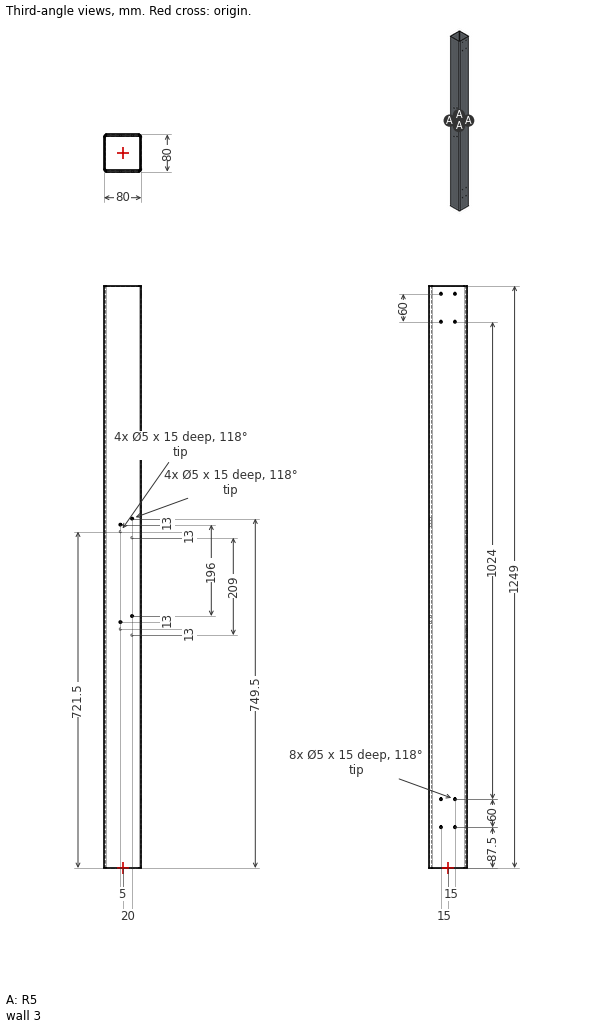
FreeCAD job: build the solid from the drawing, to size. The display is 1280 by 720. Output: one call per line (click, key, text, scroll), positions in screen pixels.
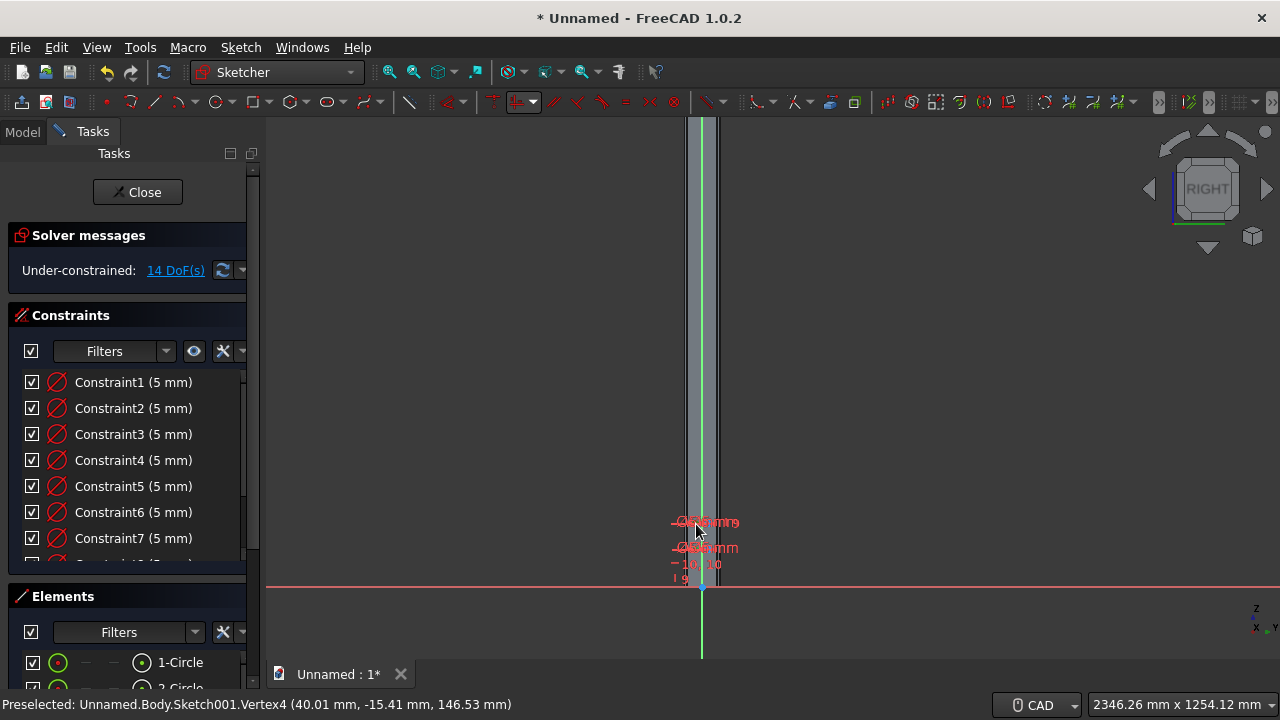
key(v)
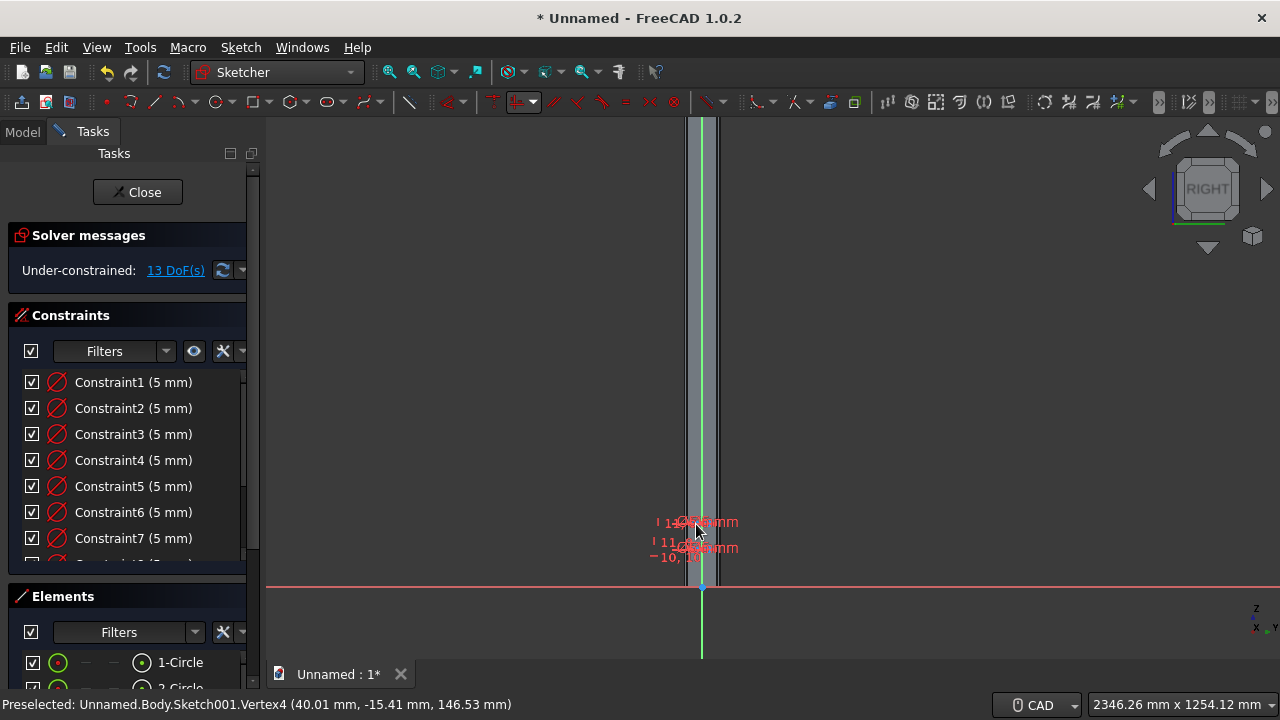
click(709, 524)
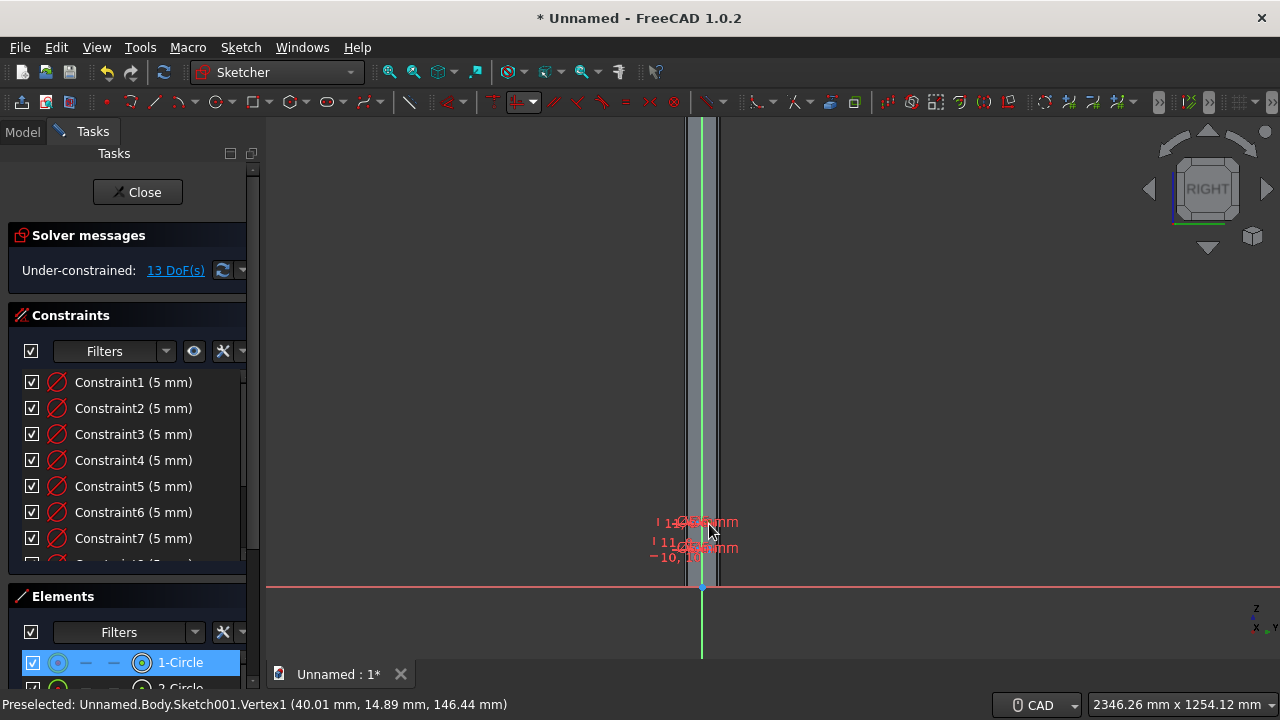
click(698, 526)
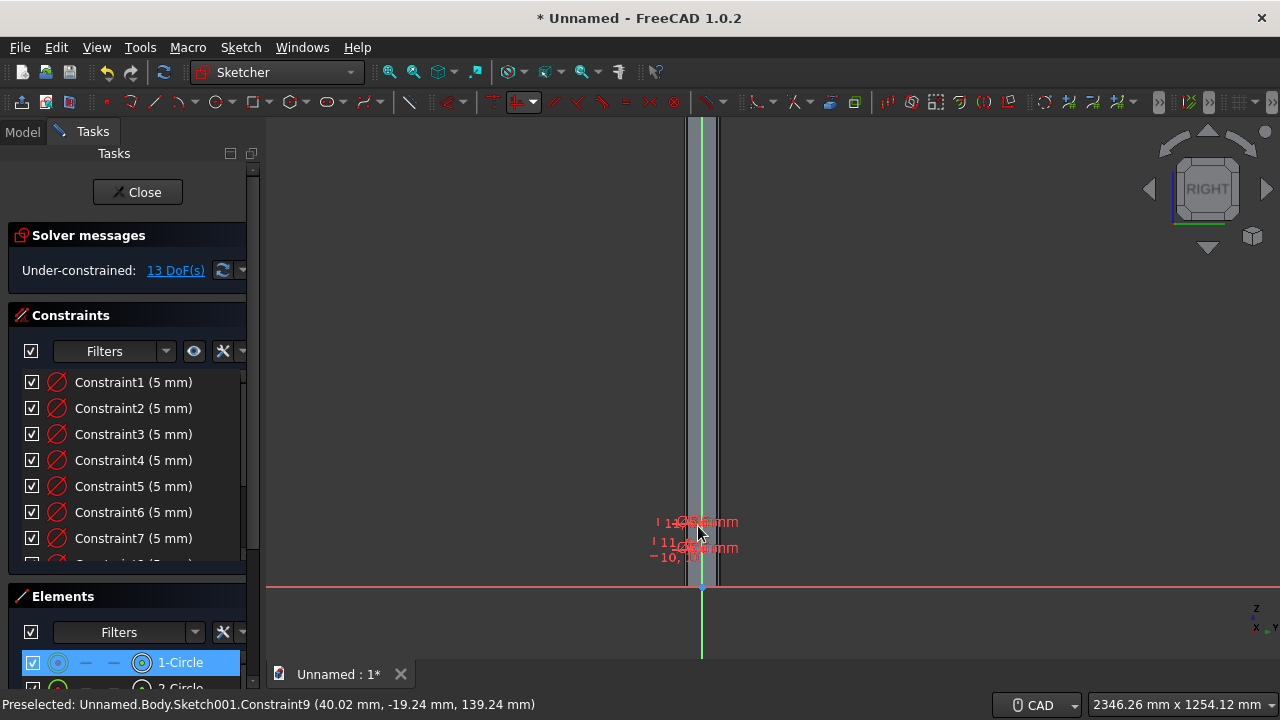
key(h)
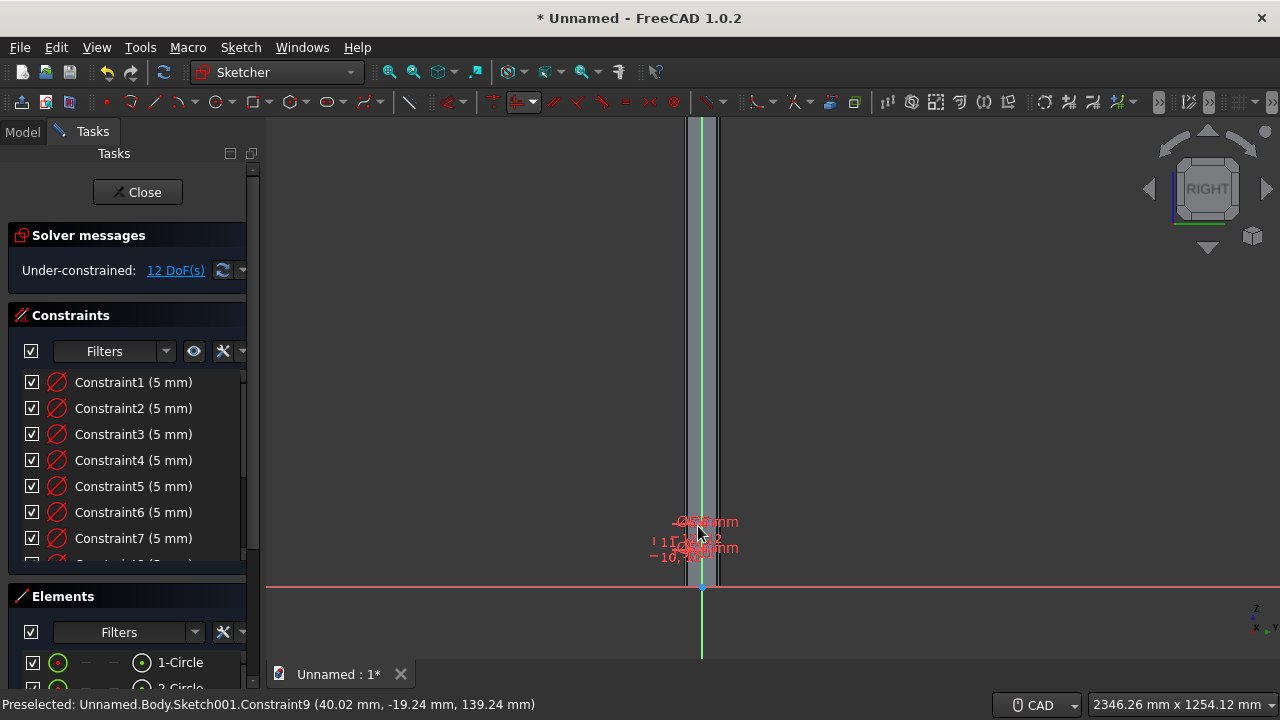
click(709, 524)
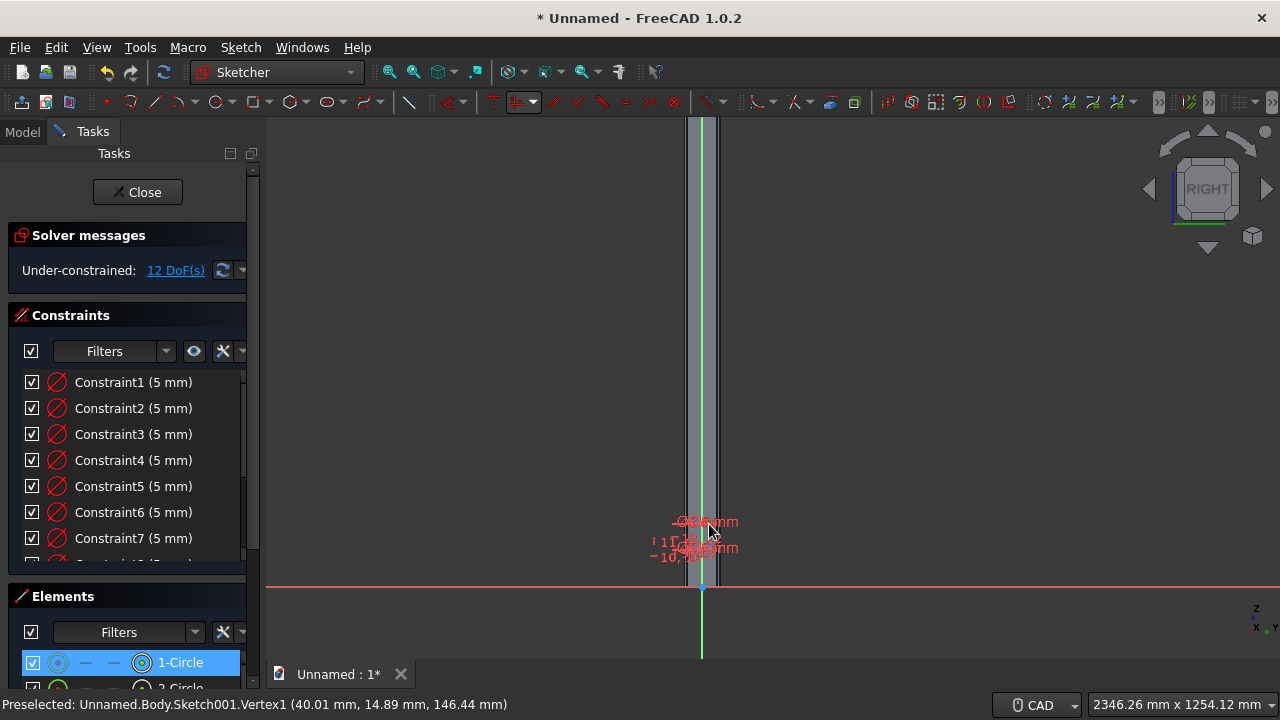
scroll(709, 525, down, 2)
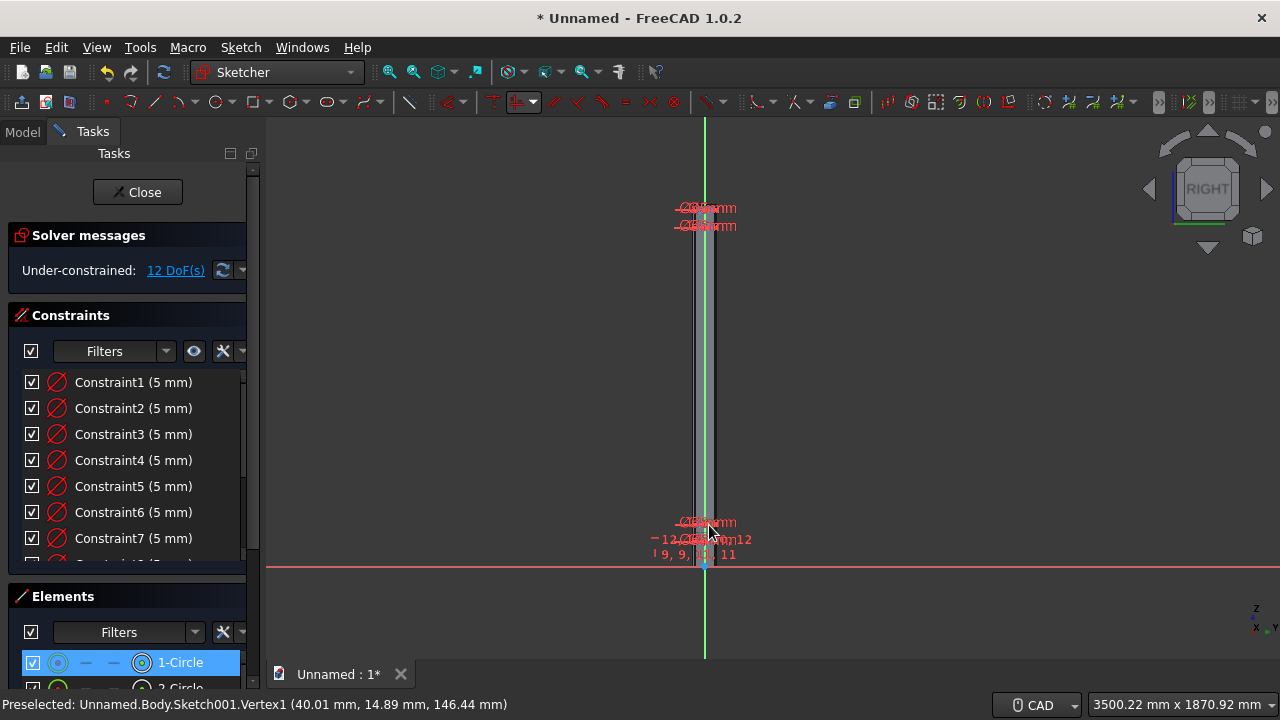
scroll(709, 228, up, 2)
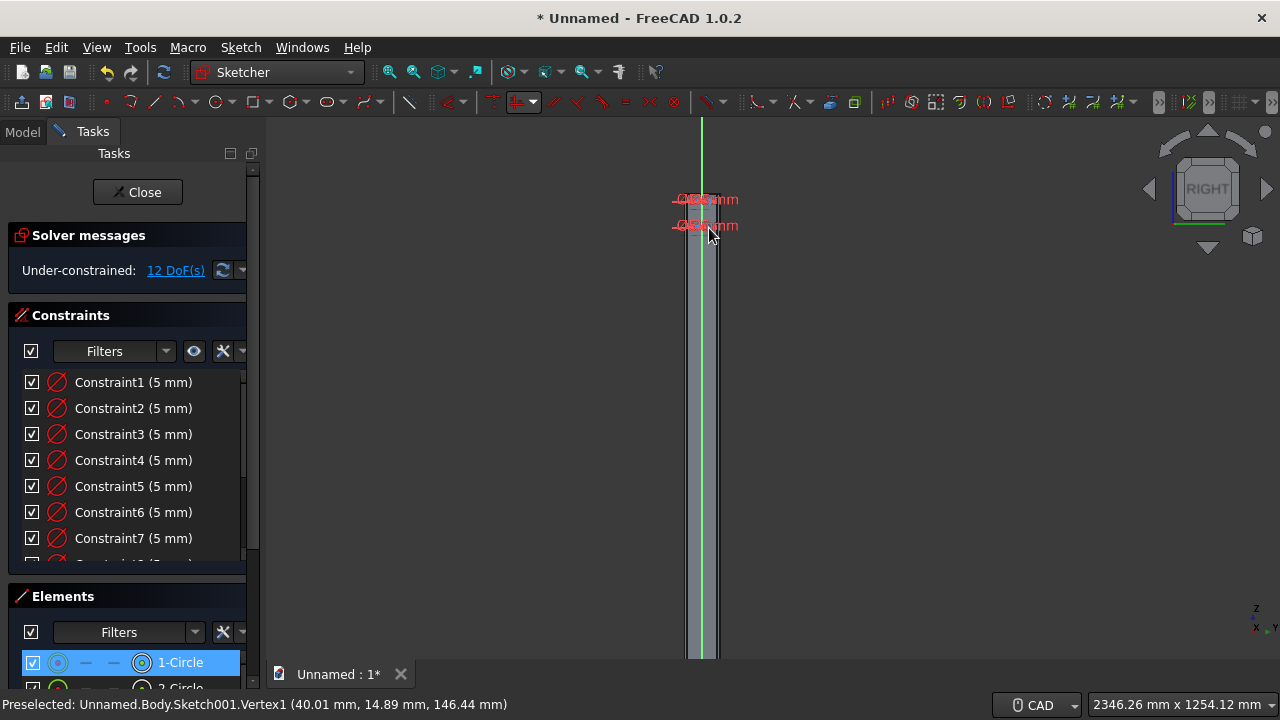
click(709, 228)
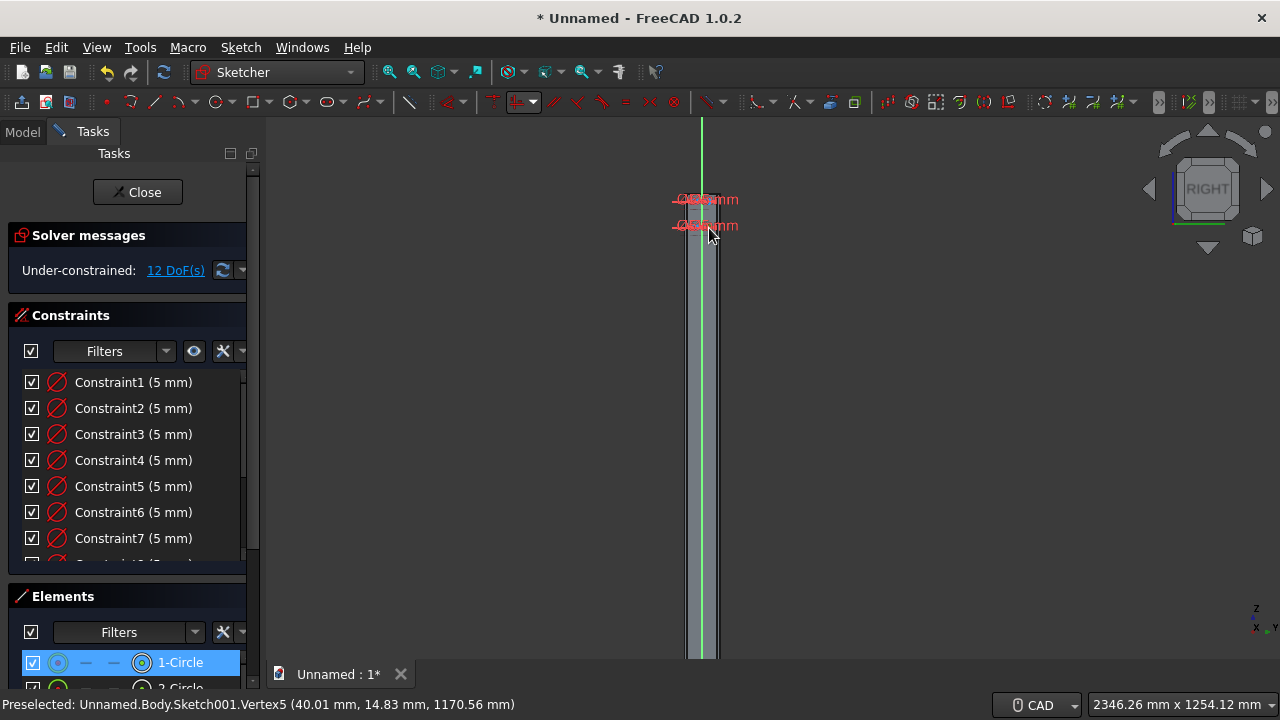
key(v)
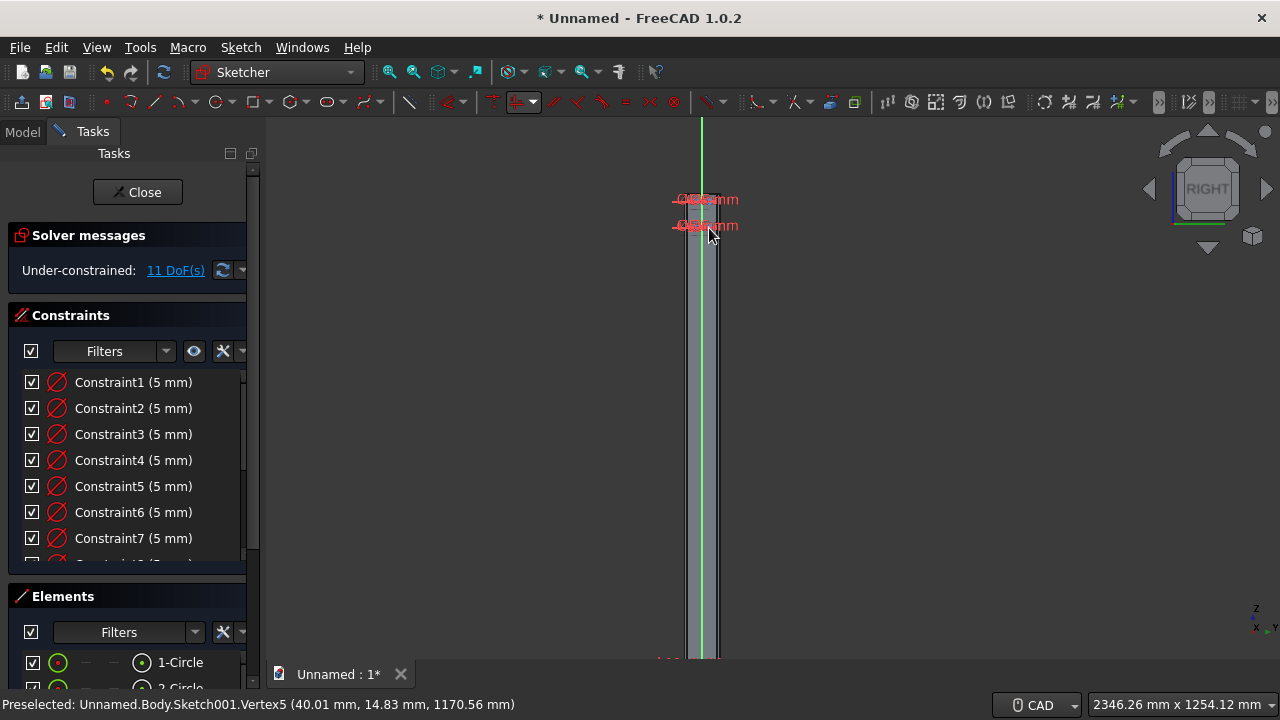
scroll(709, 228, down, 2)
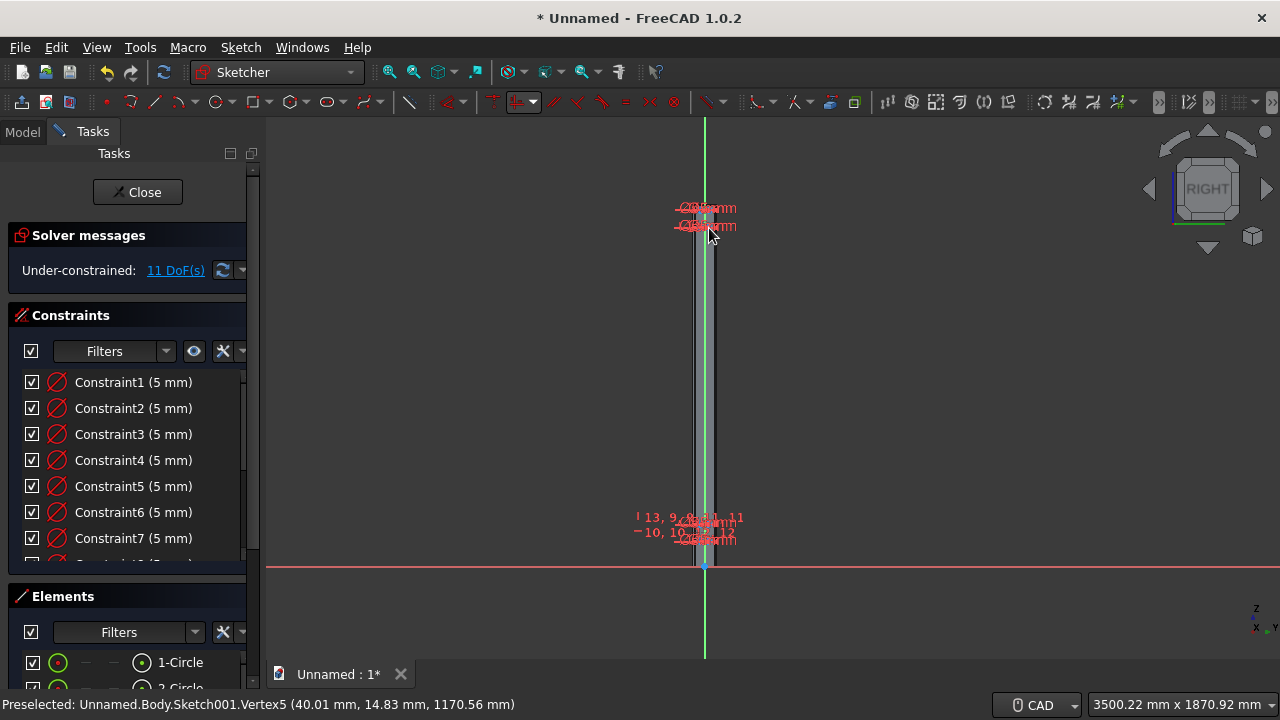
scroll(700, 525, up, 2)